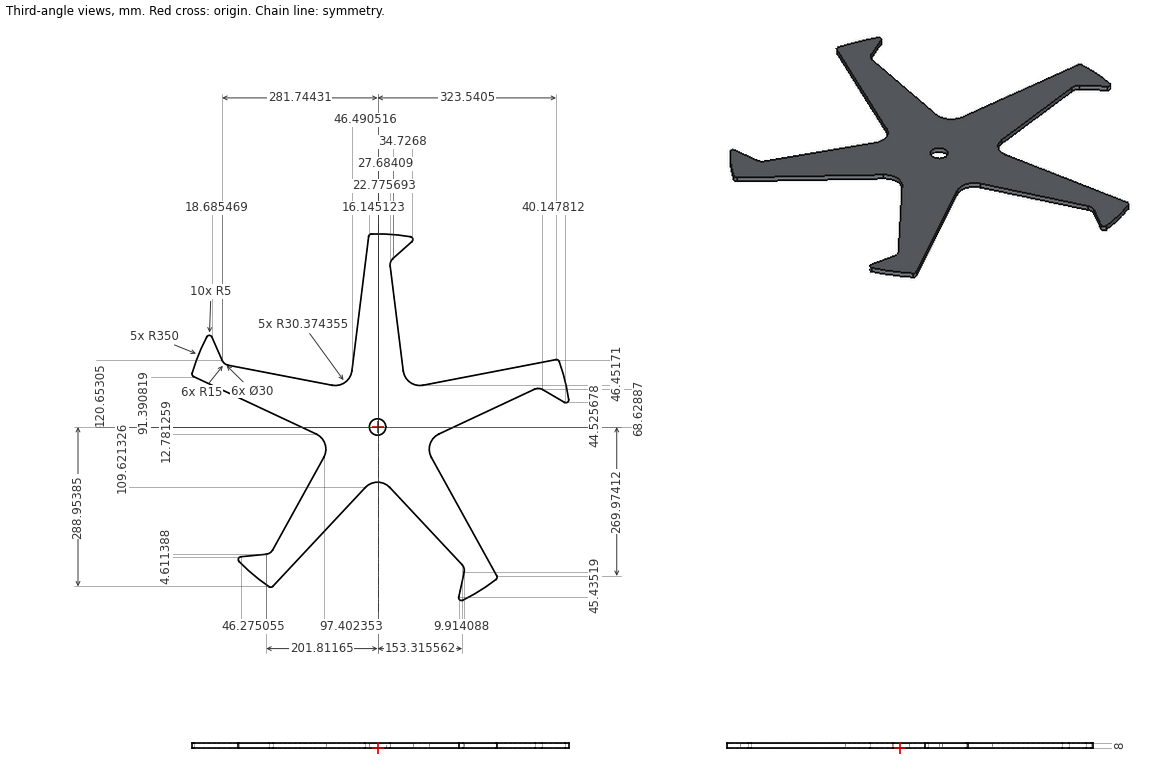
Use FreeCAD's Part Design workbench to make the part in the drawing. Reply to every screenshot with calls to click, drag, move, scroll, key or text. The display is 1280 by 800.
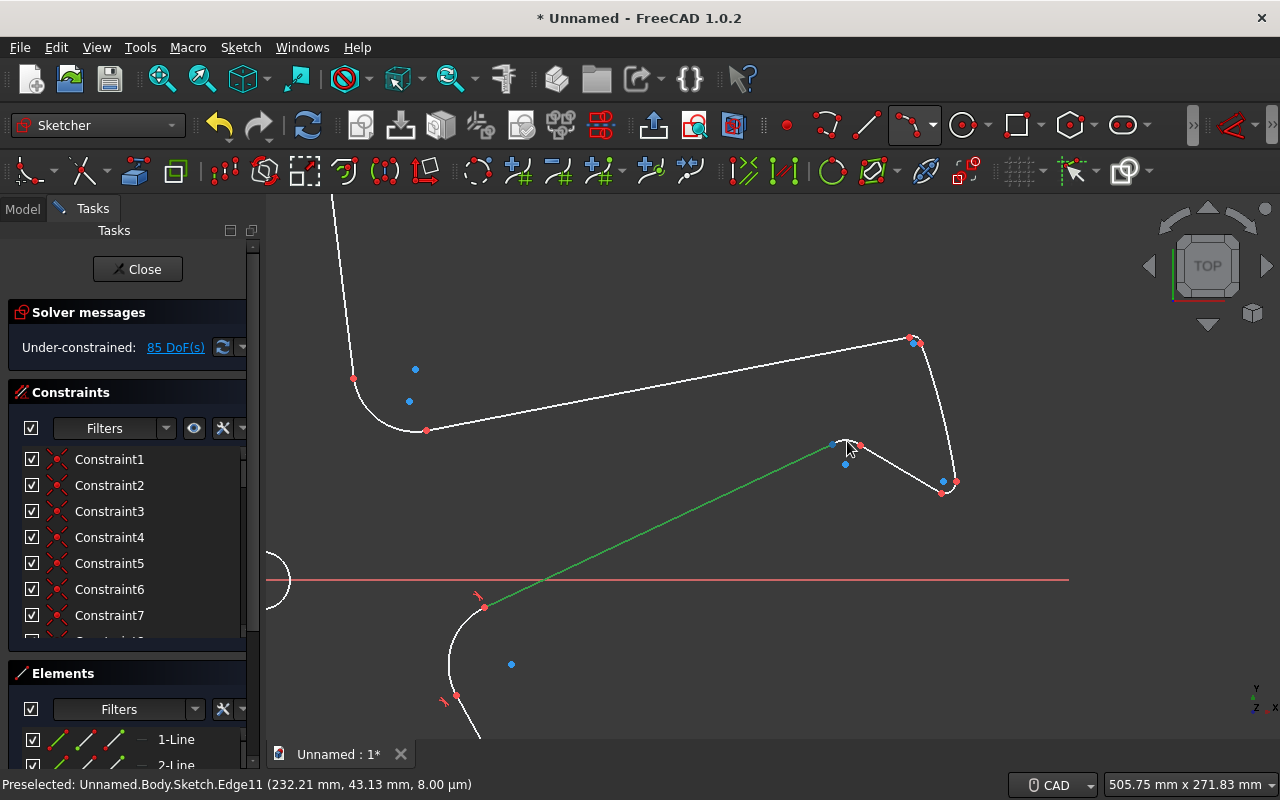
click(847, 440)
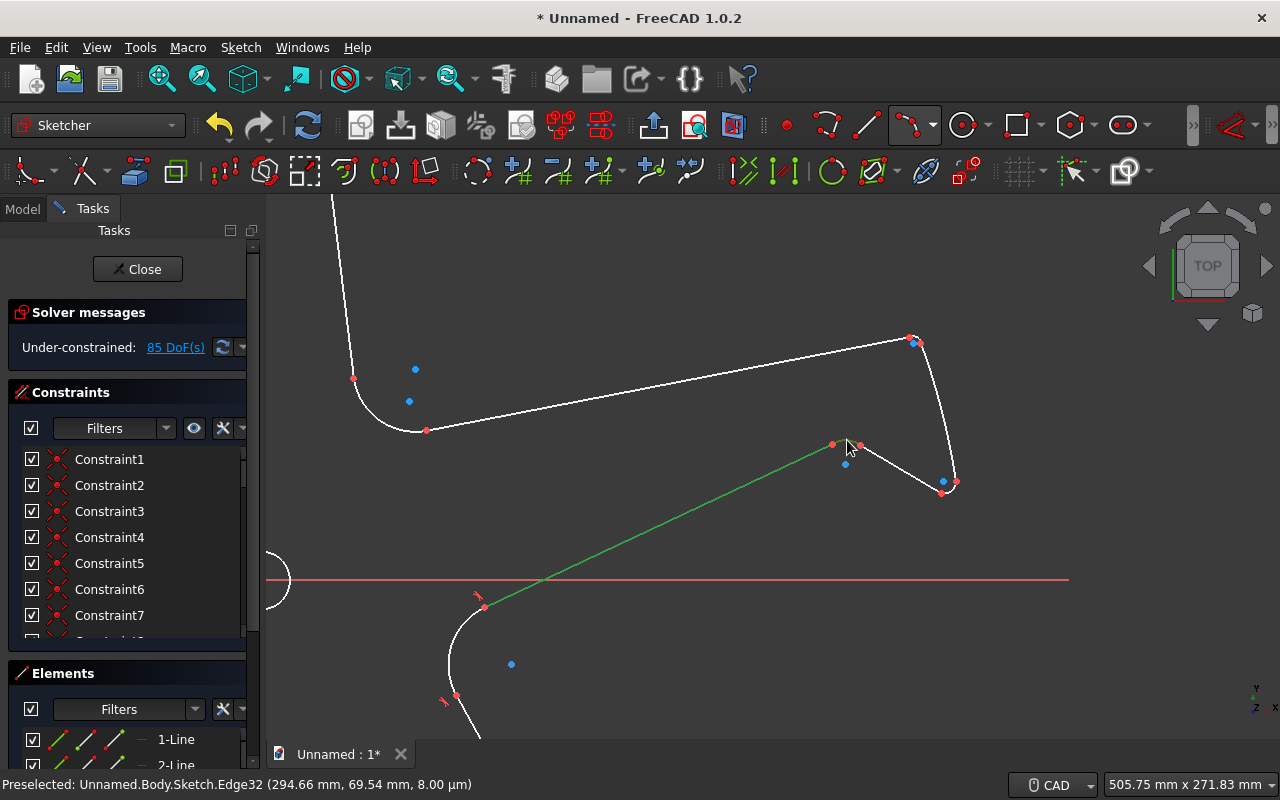
key(t)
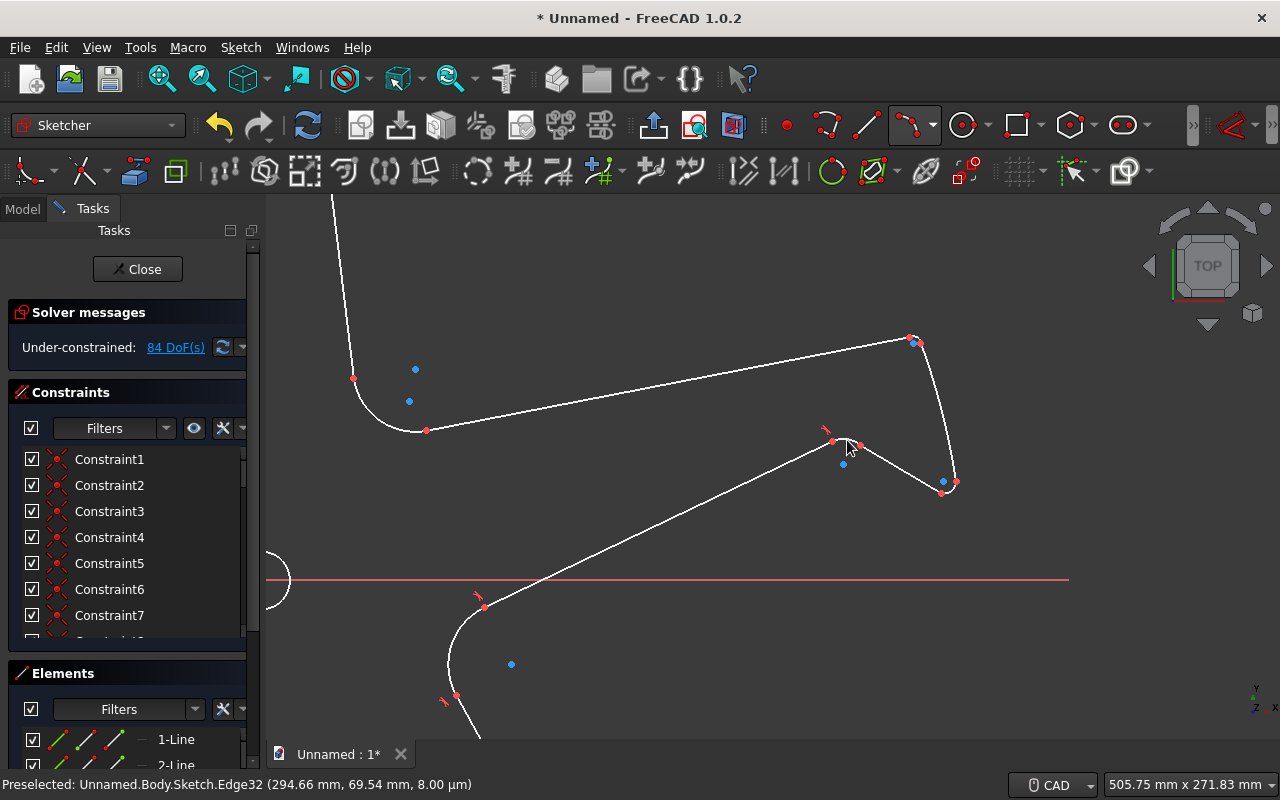
click(885, 460)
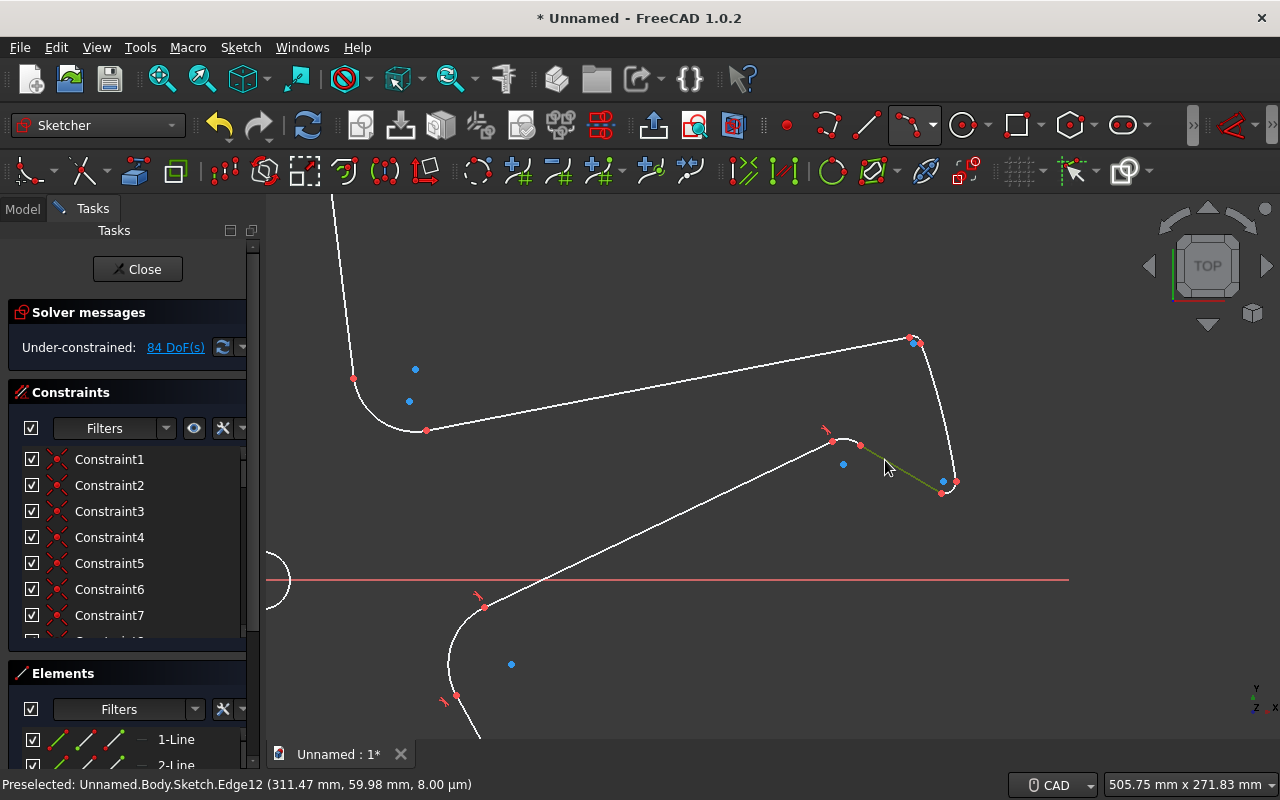
scroll(853, 441, up, 3)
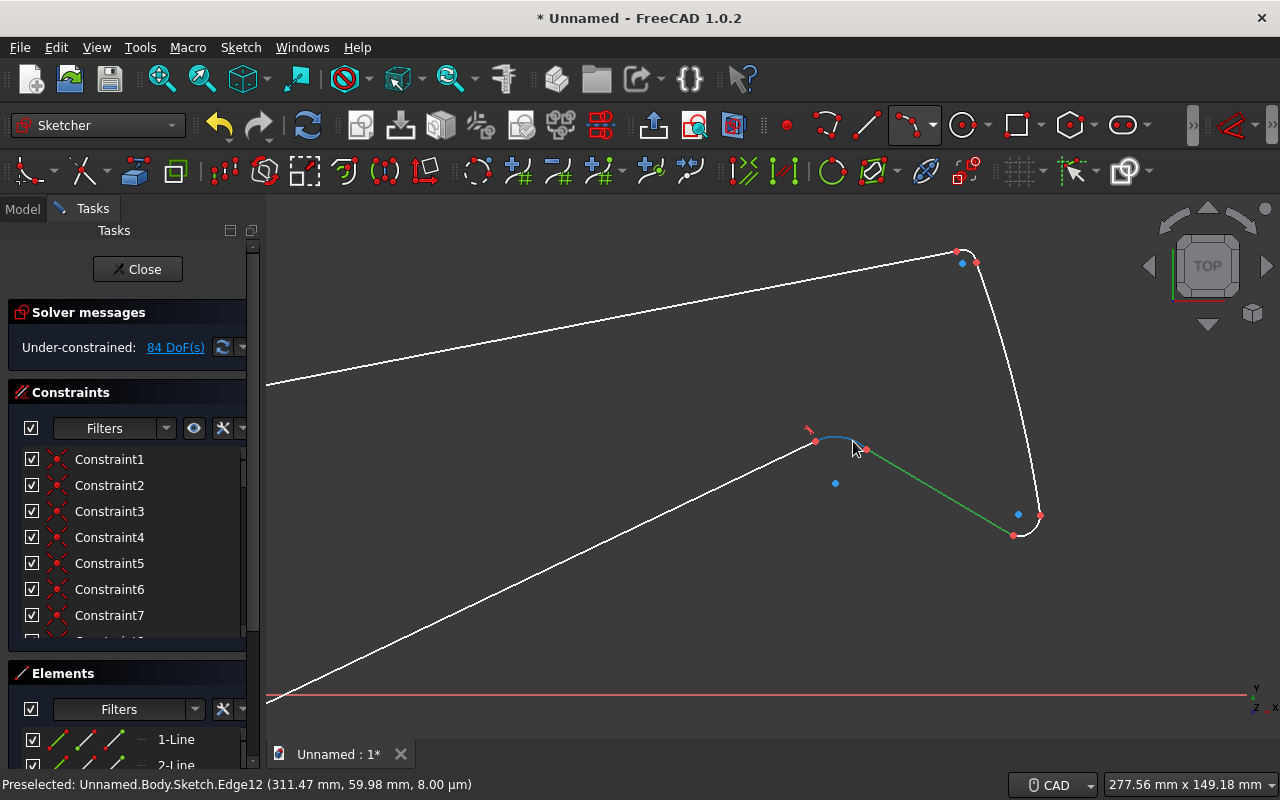
click(853, 440)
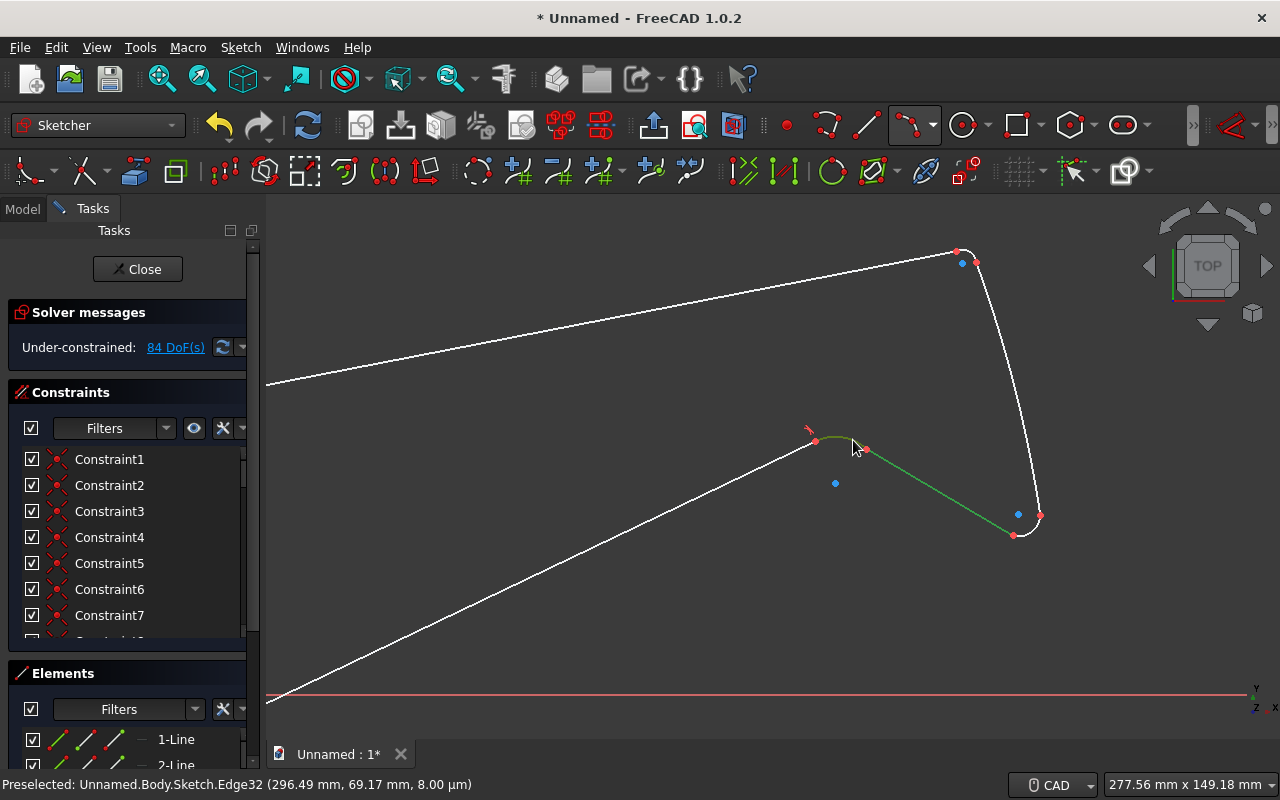
key(t)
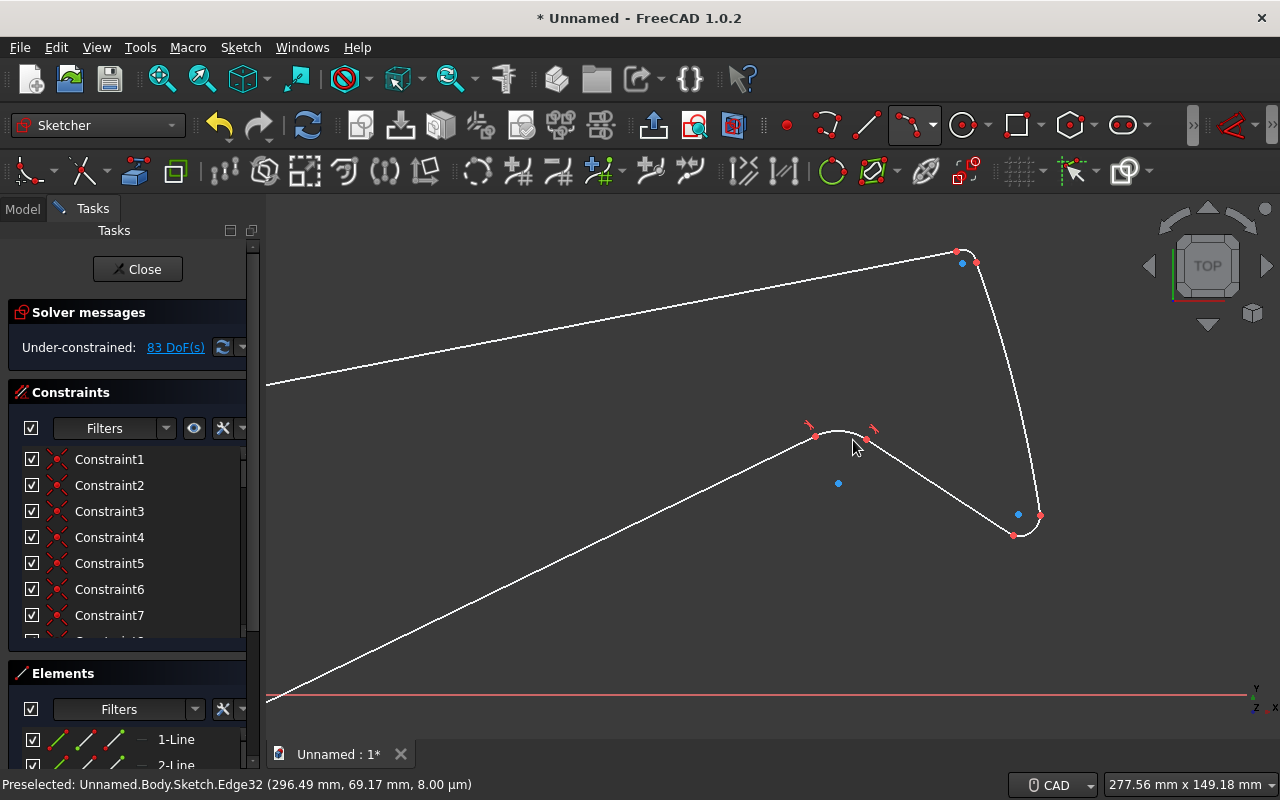
scroll(847, 441, down, 10)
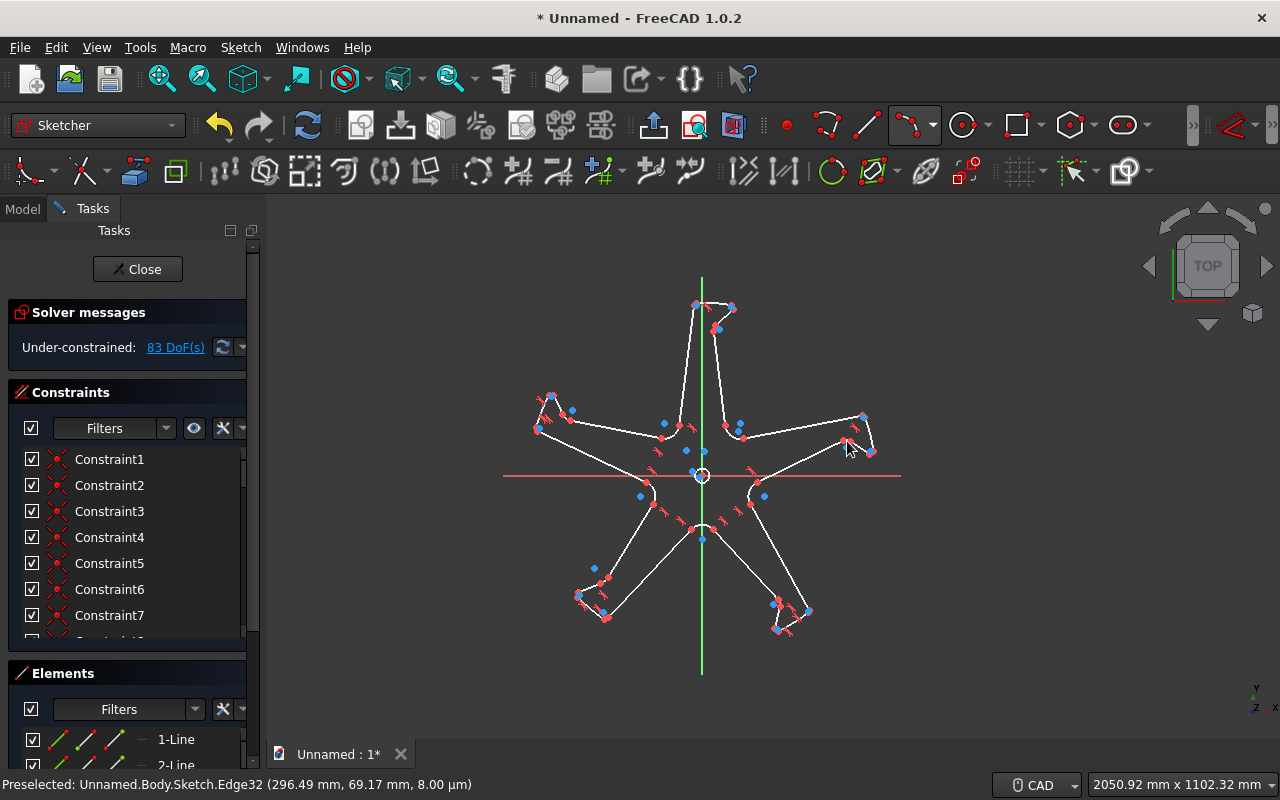
scroll(856, 445, up, 4)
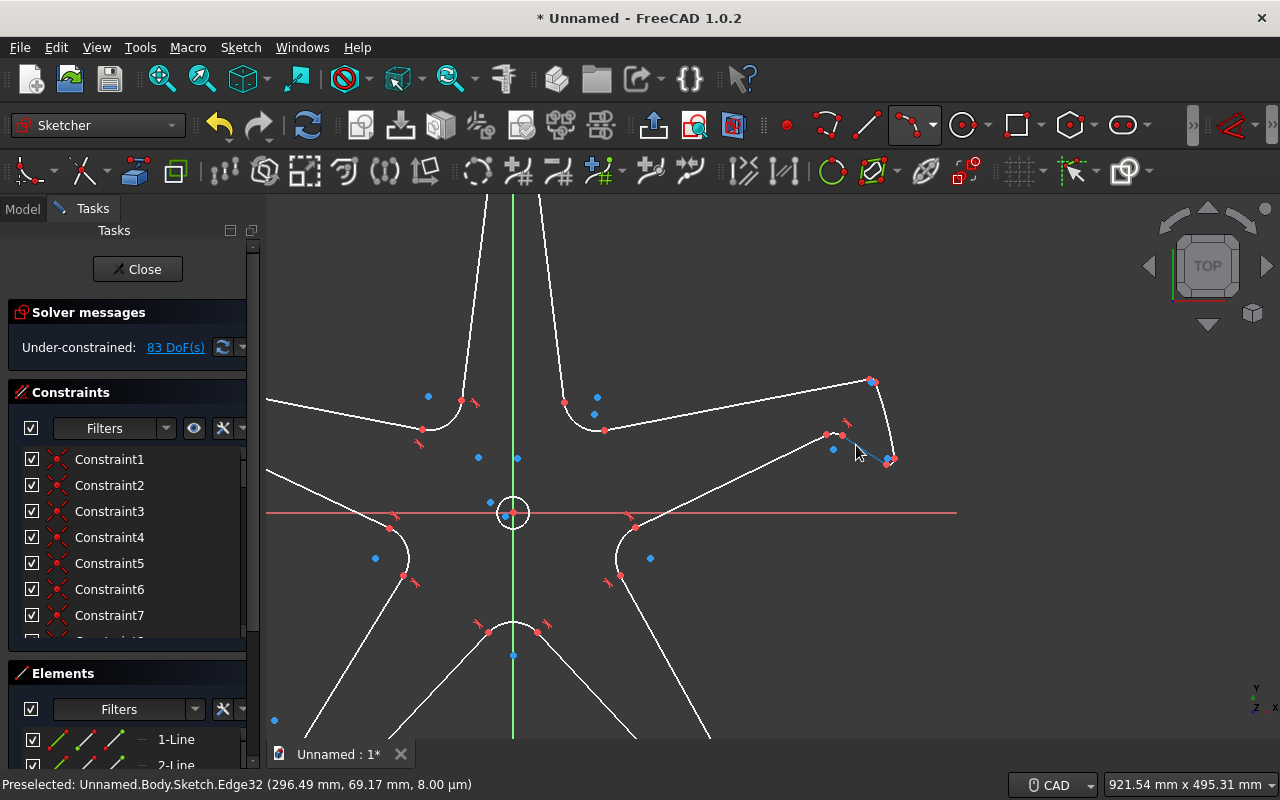
click(856, 445)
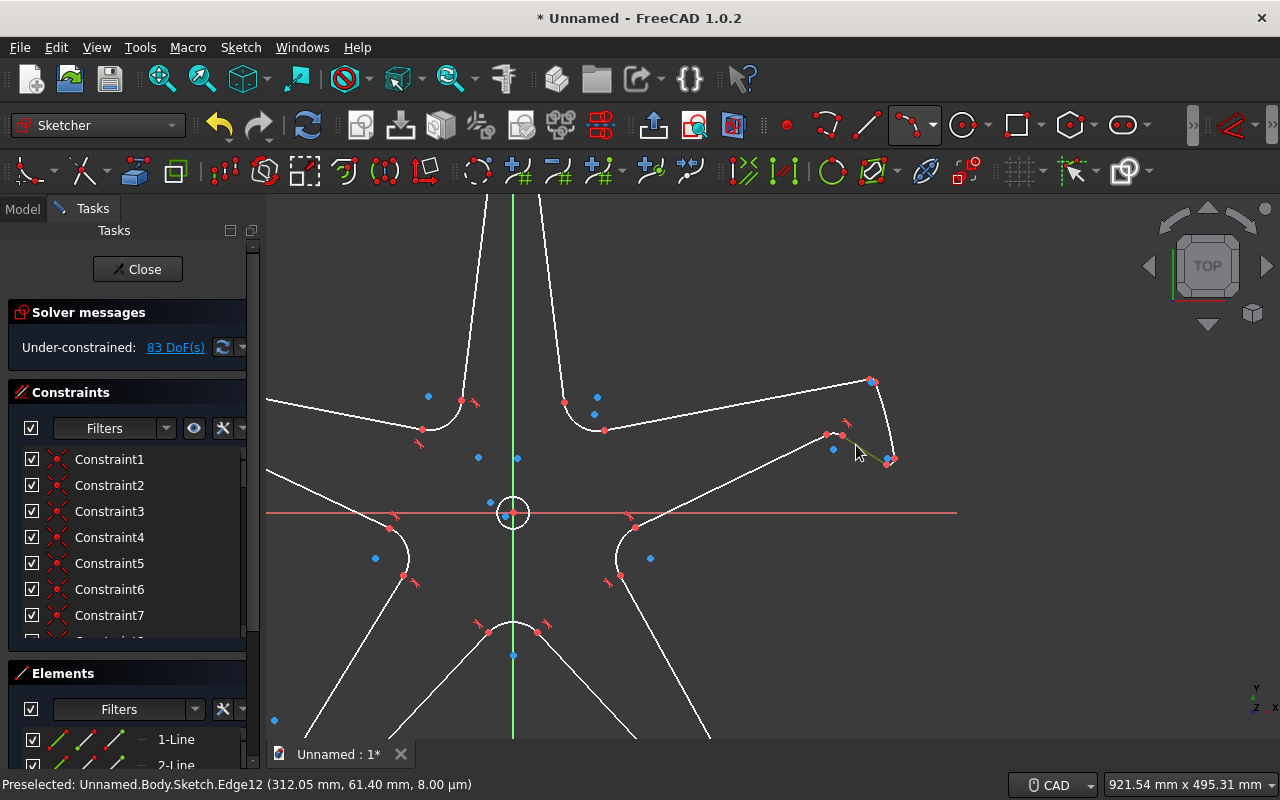
scroll(892, 464, up, 5)